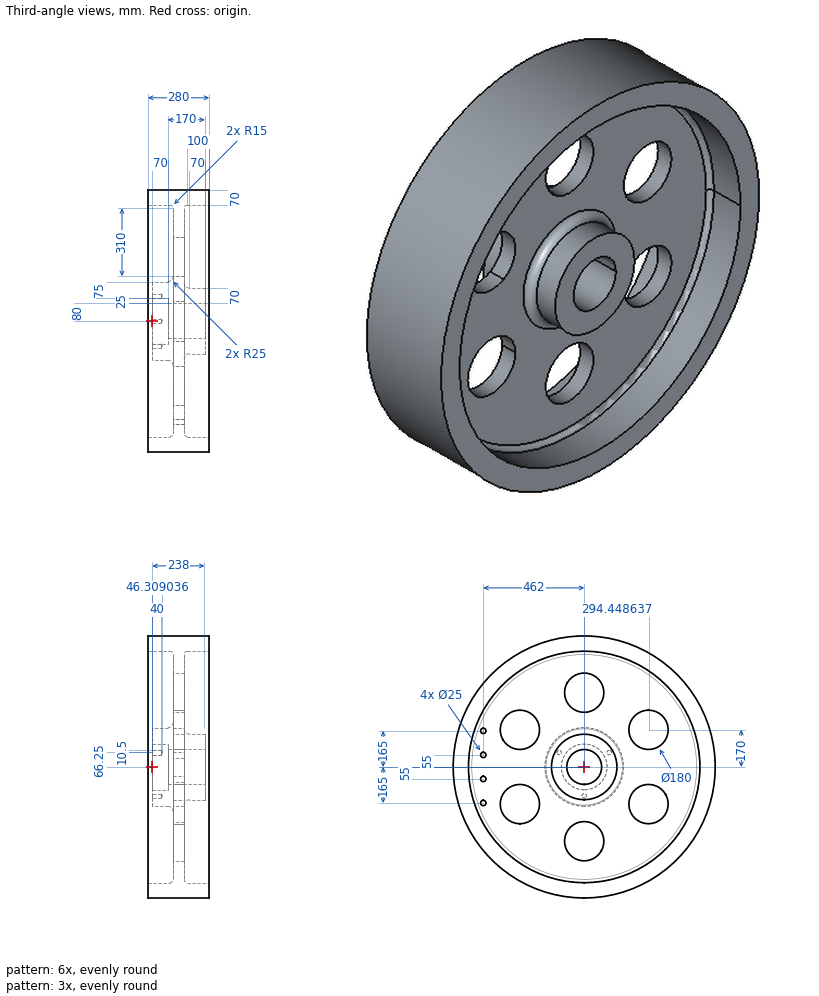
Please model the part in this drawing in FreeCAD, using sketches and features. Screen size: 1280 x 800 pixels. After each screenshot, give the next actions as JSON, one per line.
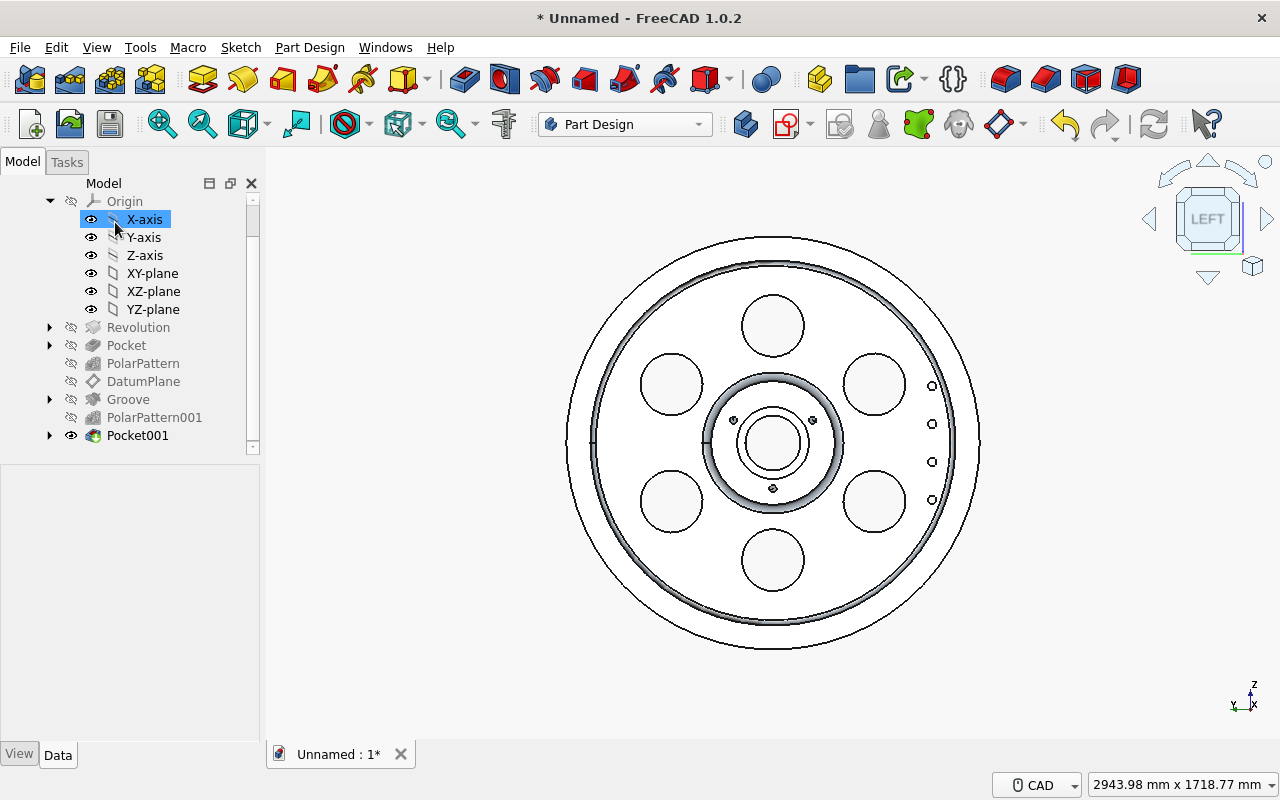
{"action": "key", "text": "0"}